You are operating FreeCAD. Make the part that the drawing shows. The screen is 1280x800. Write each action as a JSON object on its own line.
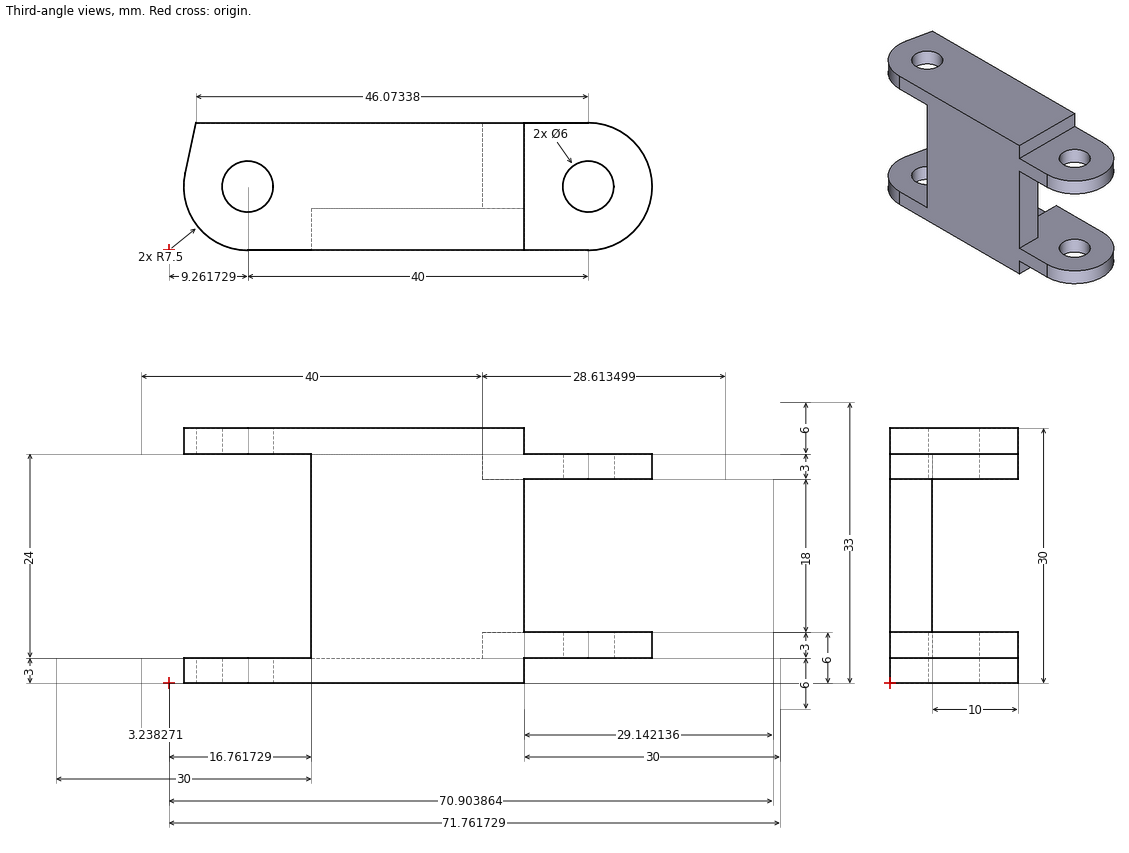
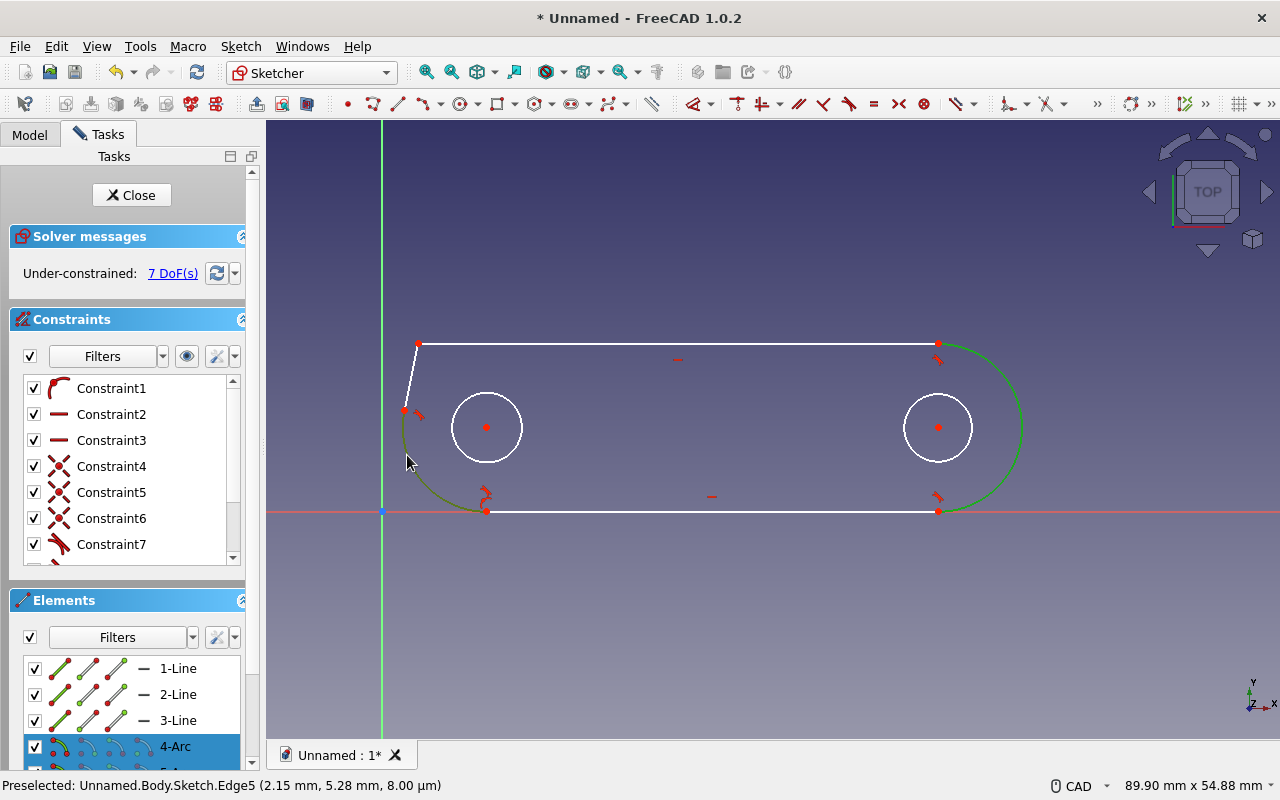
{"action": "left_click", "coordinate": [874, 104]}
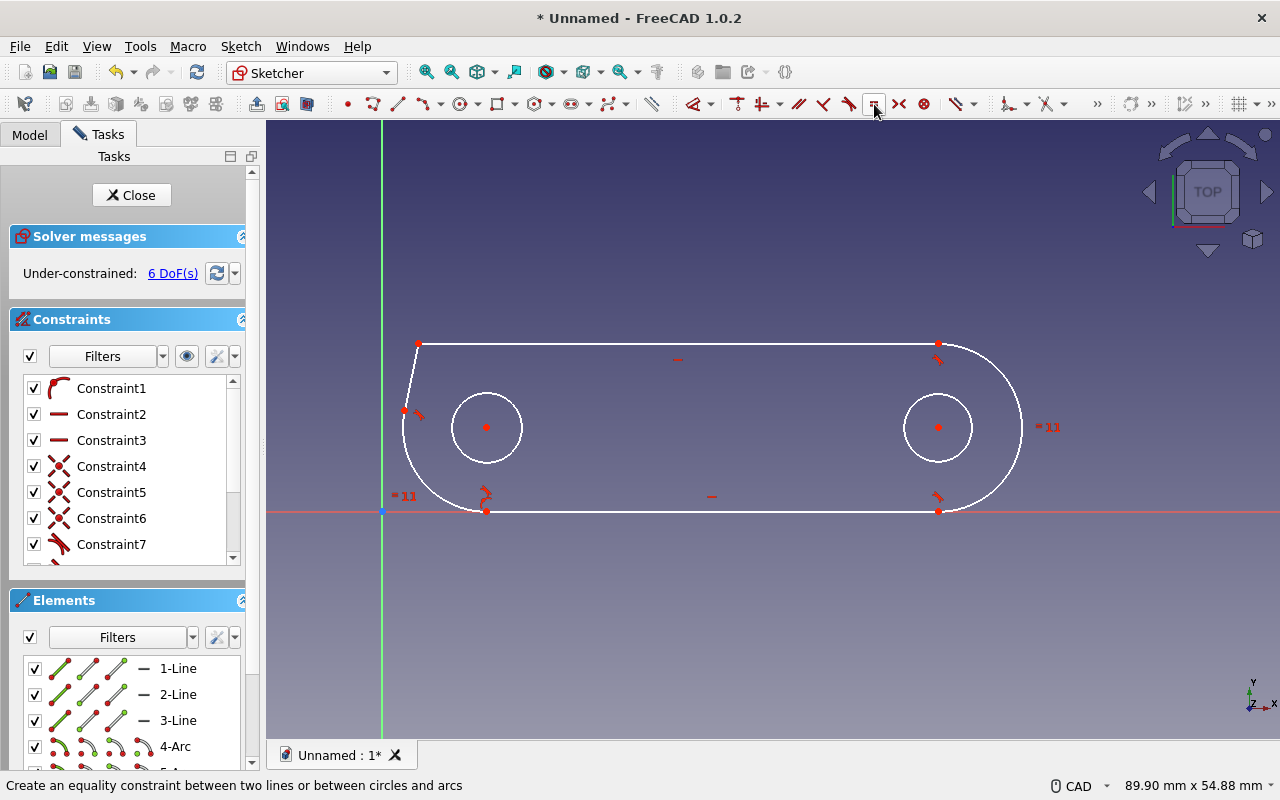
{"action": "left_click", "coordinate": [962, 404]}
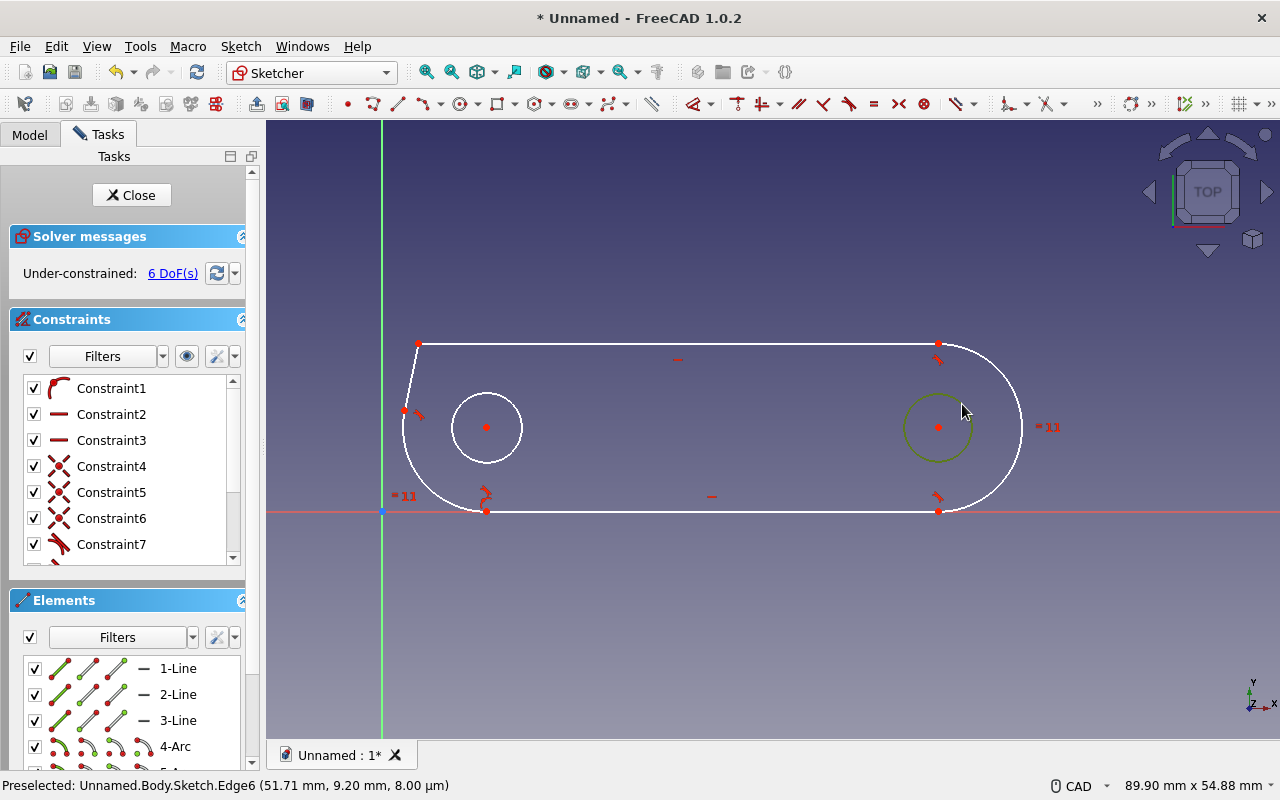
{"action": "left_click", "coordinate": [512, 403]}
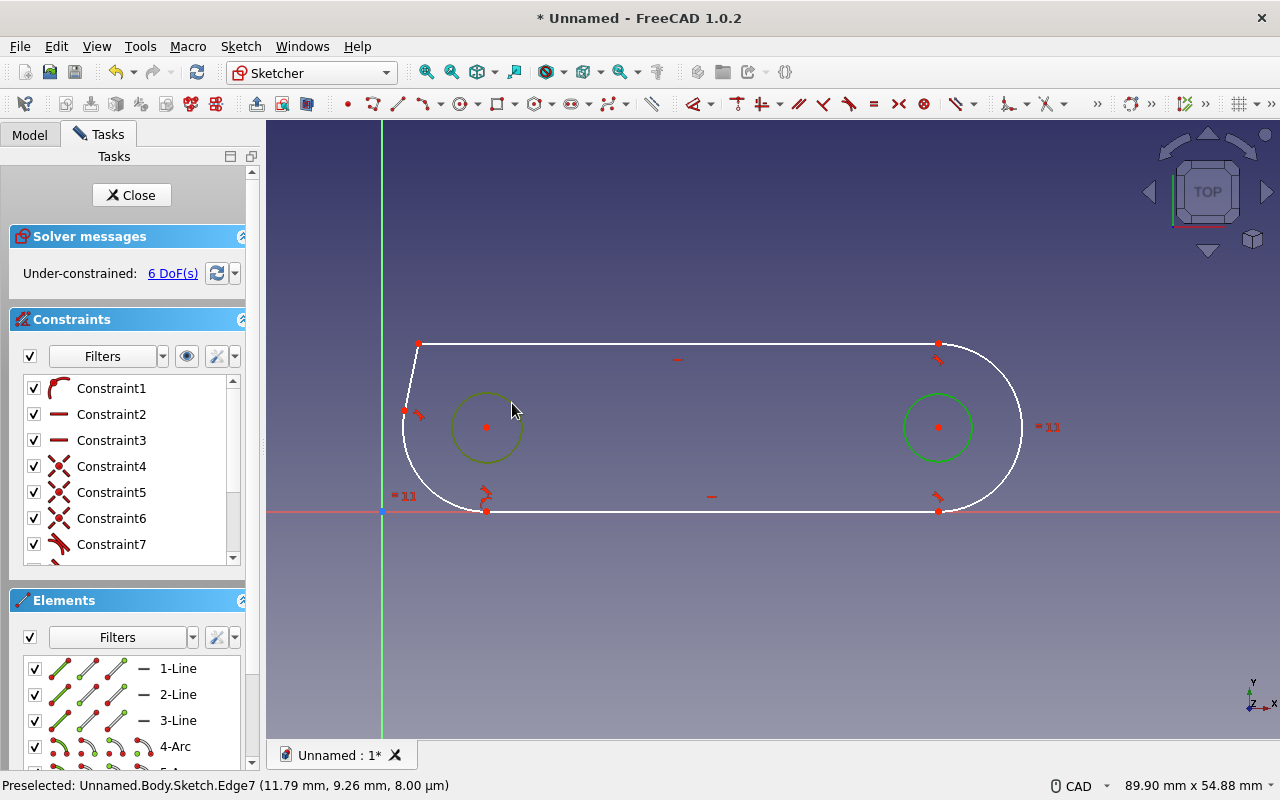
{"action": "left_click", "coordinate": [874, 104]}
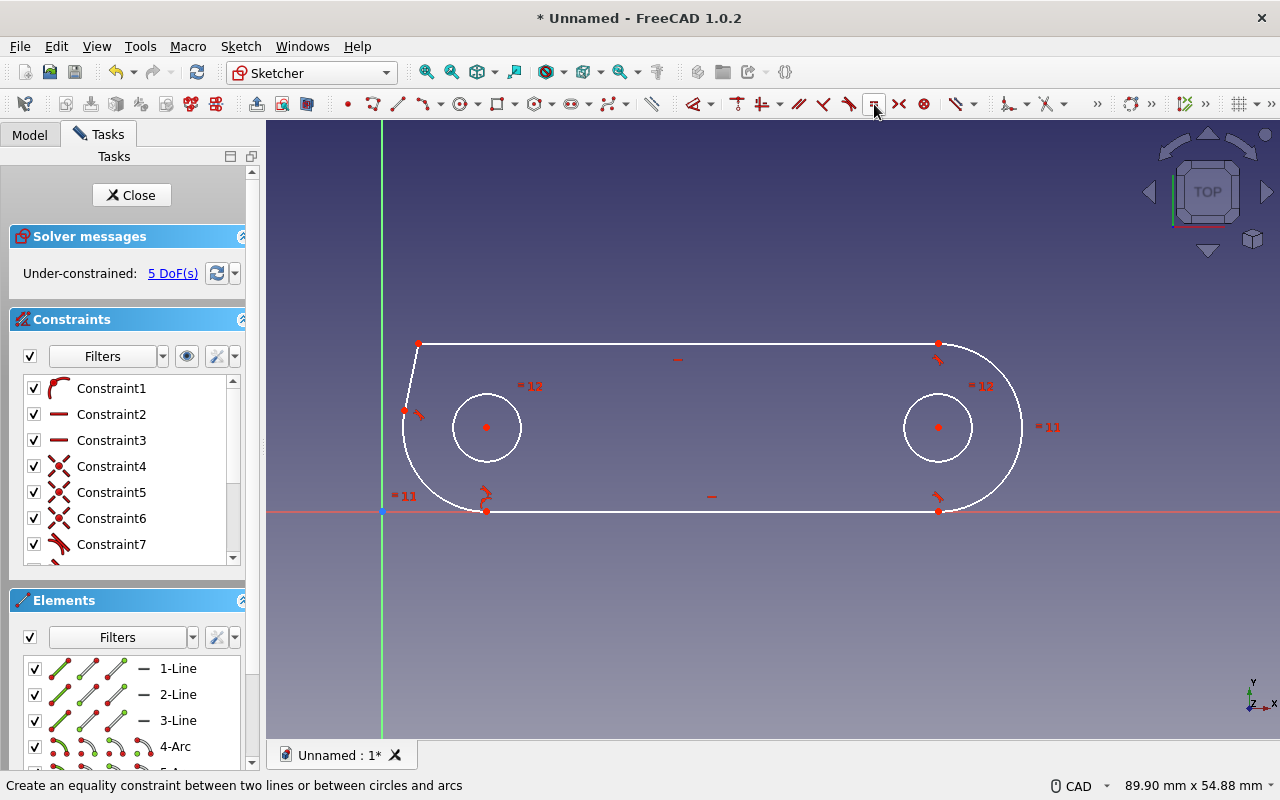
{"action": "left_click", "coordinate": [692, 104]}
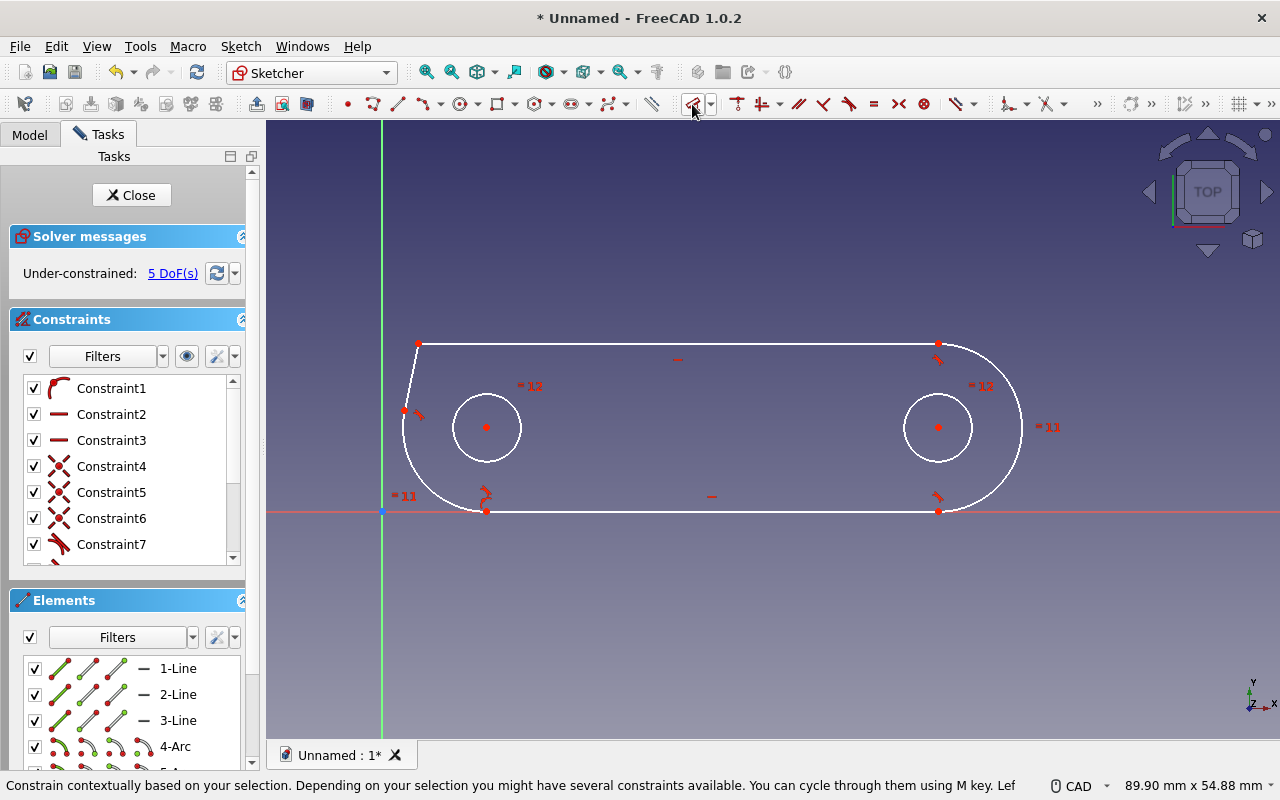
{"action": "left_click", "coordinate": [1006, 477]}
{"action": "left_click", "coordinate": [1032, 496]}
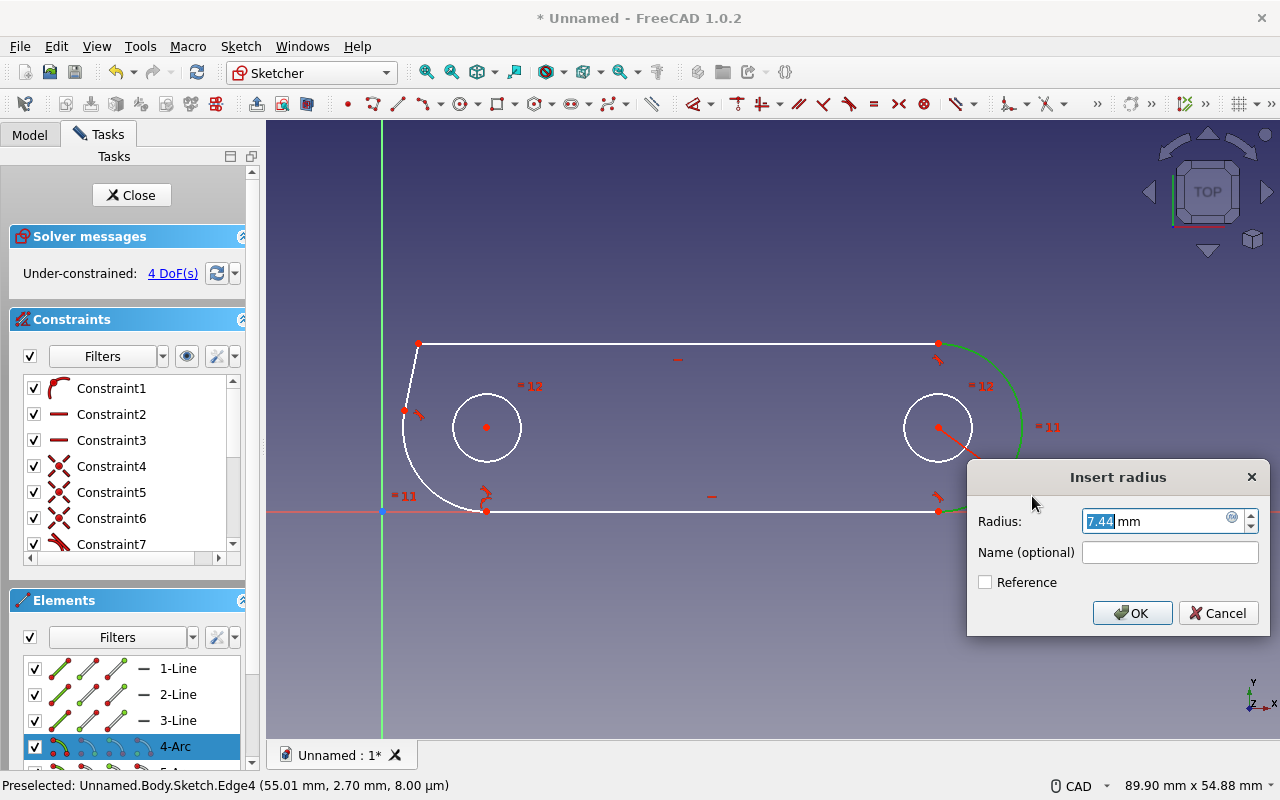
{"action": "type", "text": "7.5"}
{"action": "key", "text": "Return"}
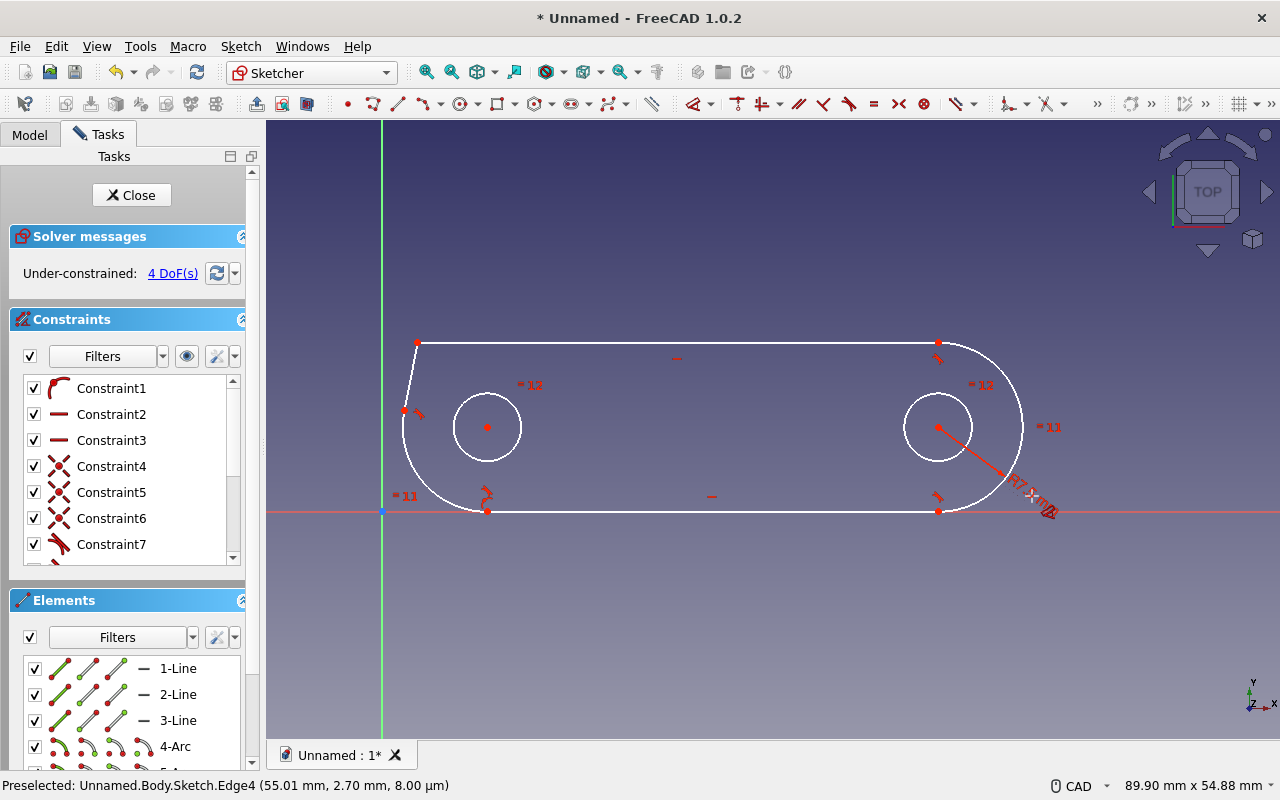
{"action": "left_click", "coordinate": [962, 403]}
{"action": "left_click", "coordinate": [984, 380]}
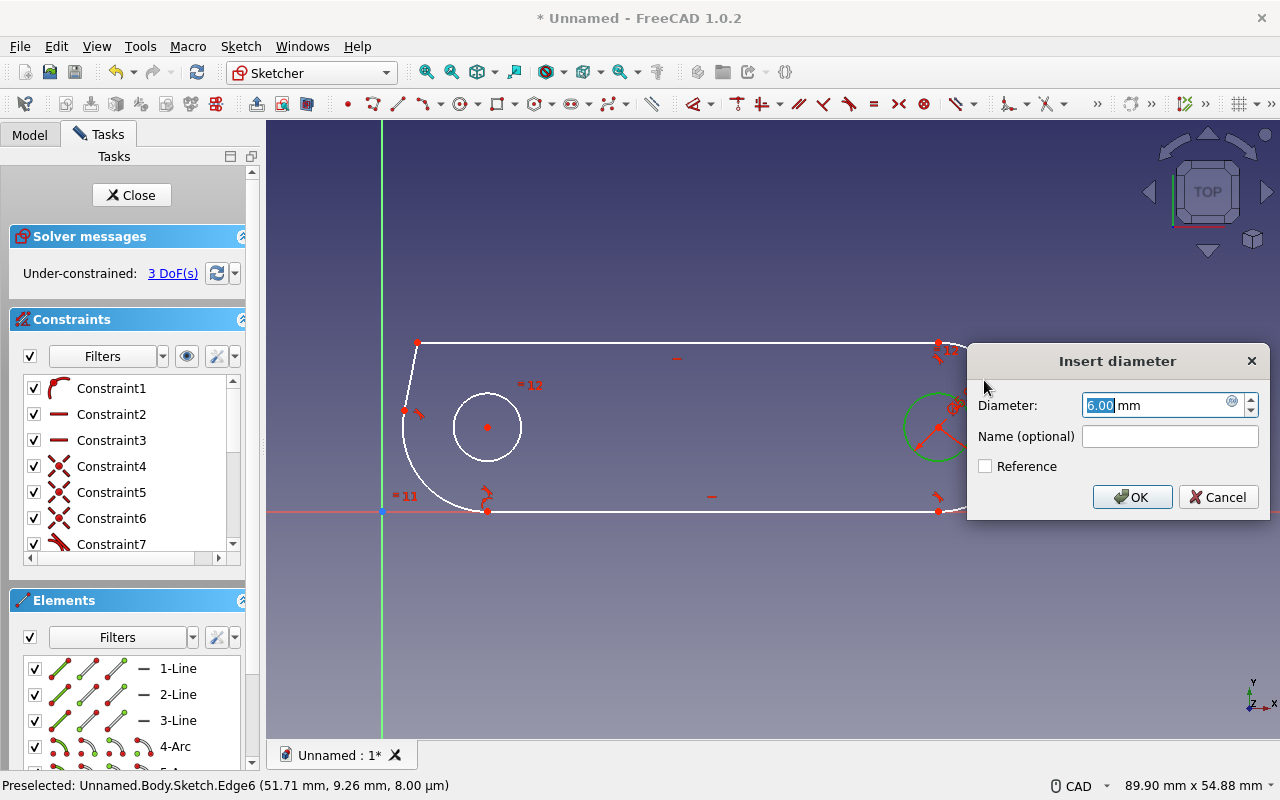
{"action": "type", "text": "6"}
{"action": "key", "text": "Return"}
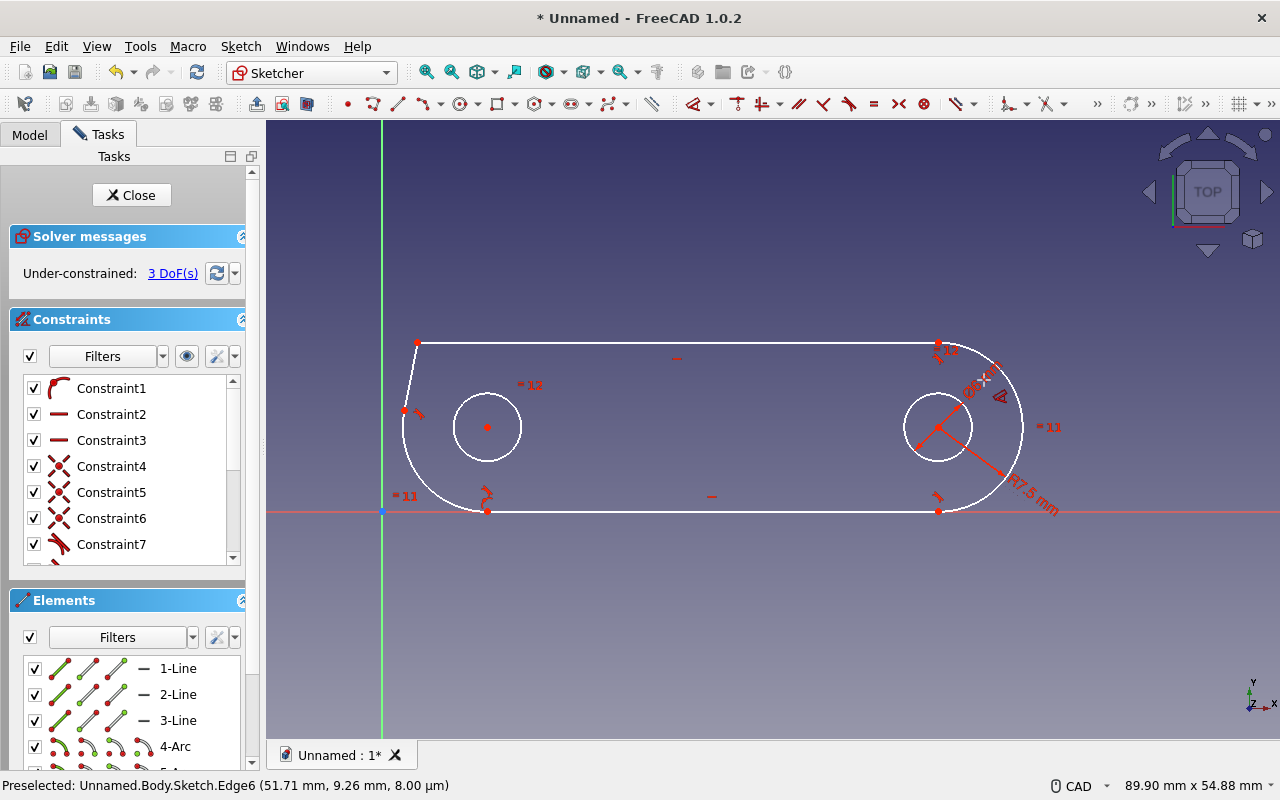
{"action": "left_click", "coordinate": [623, 512]}
{"action": "left_click", "coordinate": [713, 546]}